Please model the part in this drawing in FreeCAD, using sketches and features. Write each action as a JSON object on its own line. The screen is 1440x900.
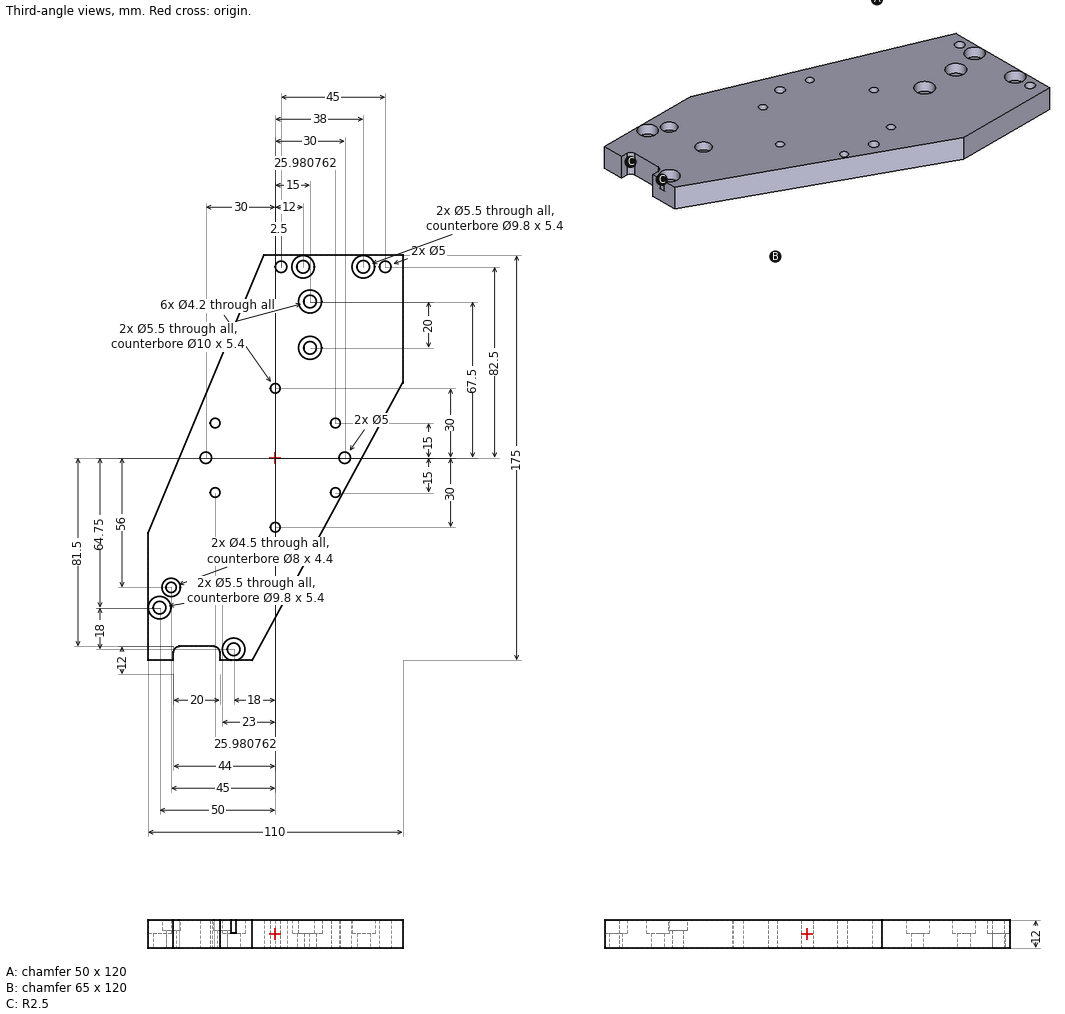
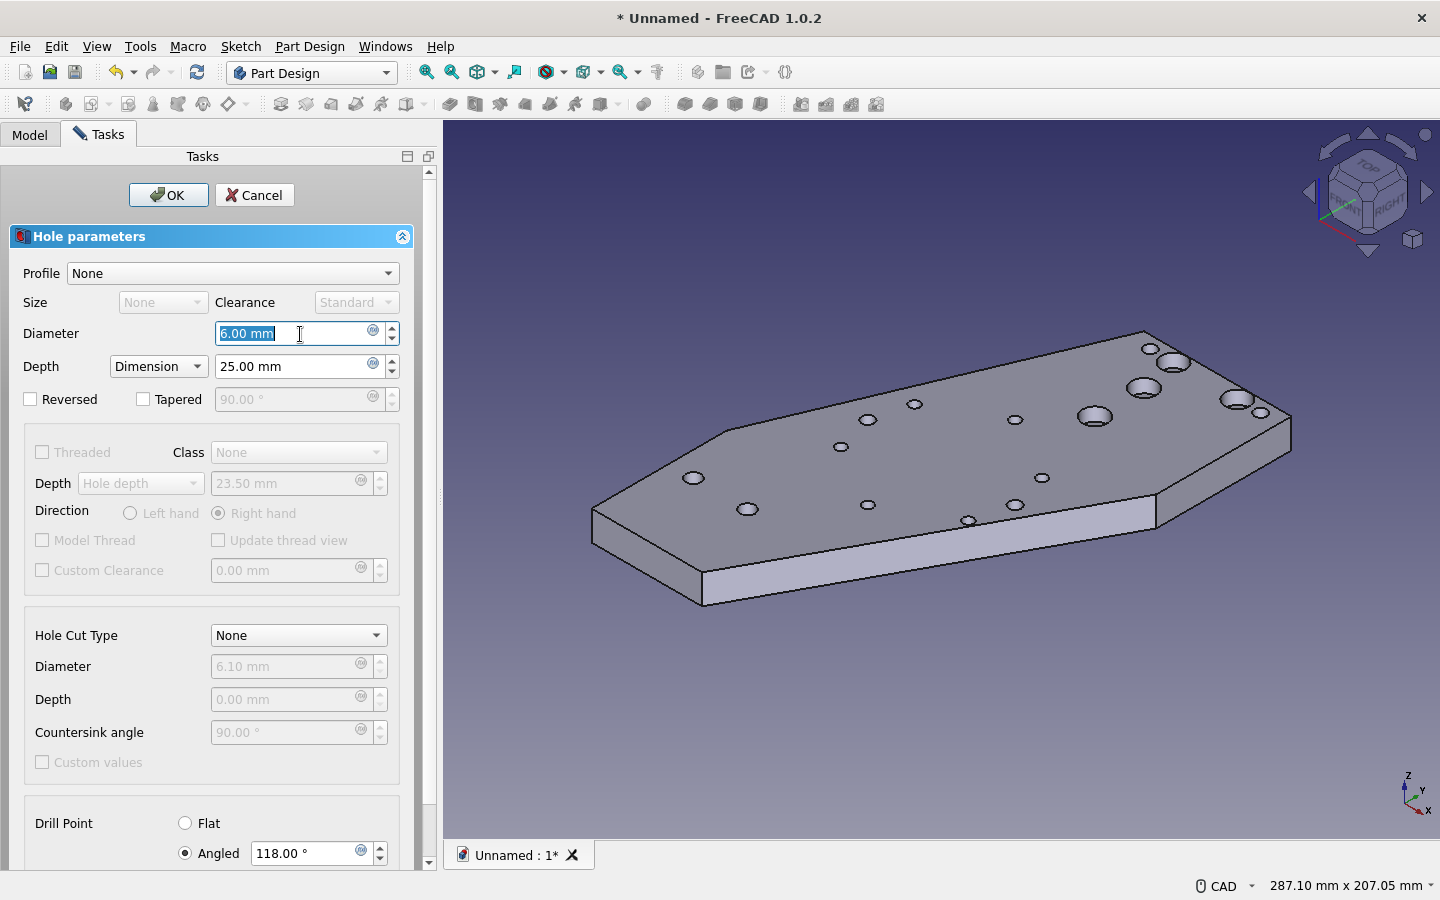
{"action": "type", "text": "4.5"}
{"action": "key", "text": "Tab"}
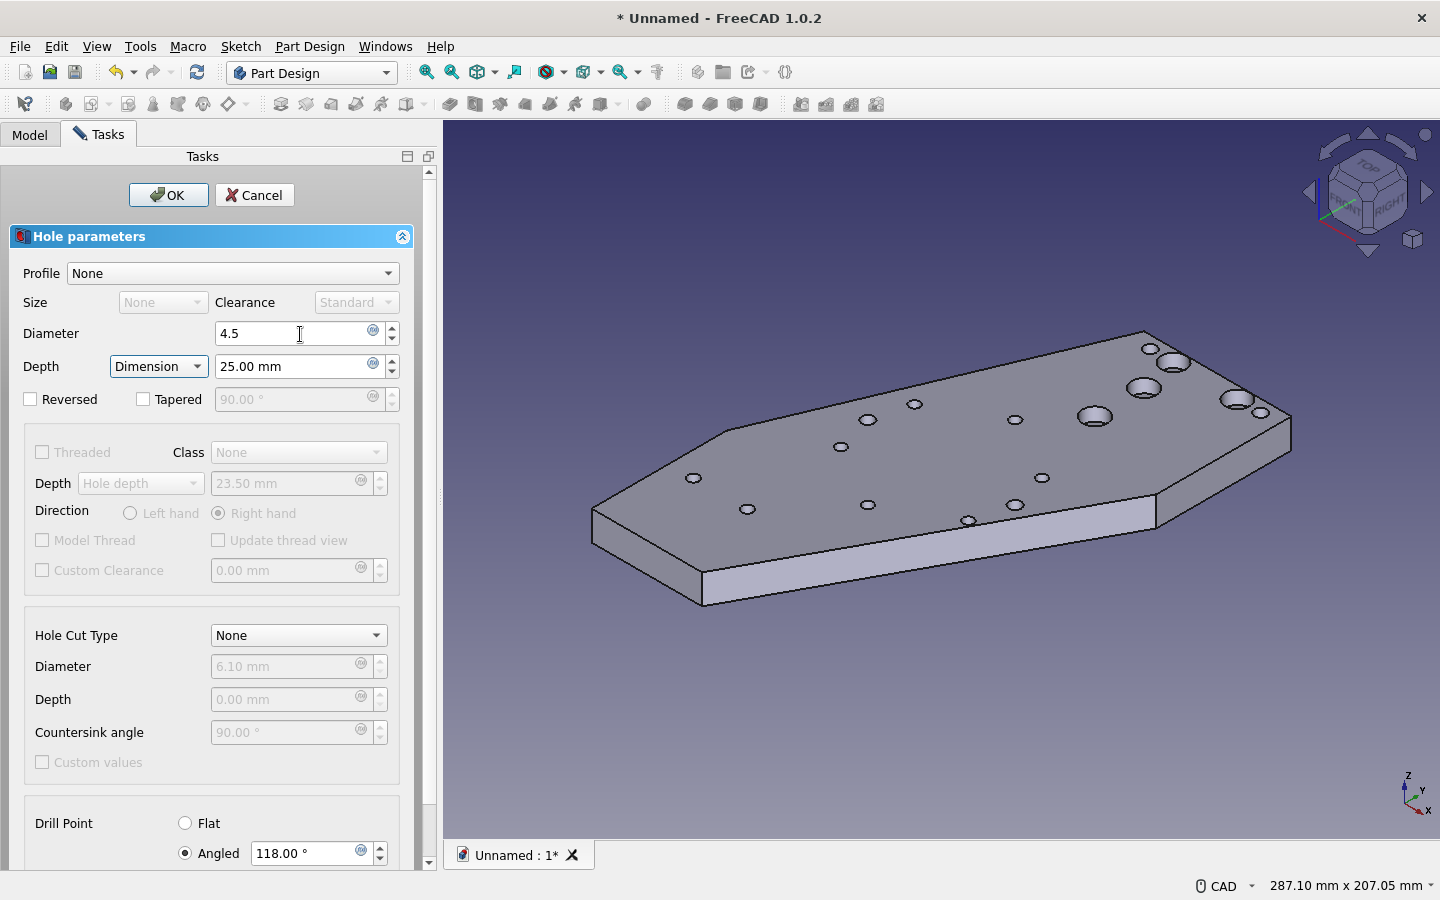
{"action": "left_click", "coordinate": [160, 366]}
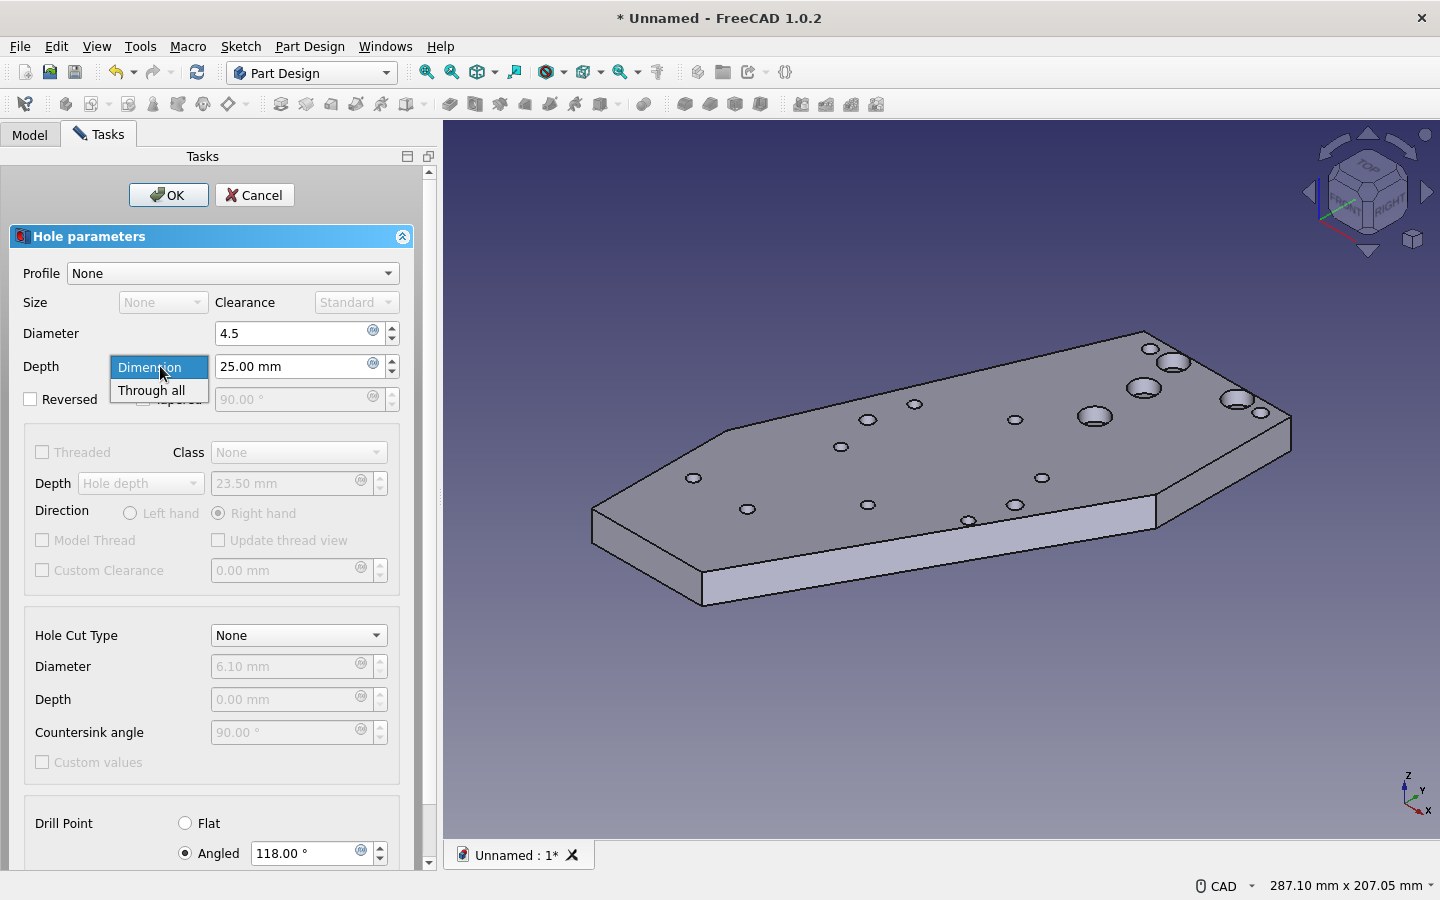
{"action": "left_click", "coordinate": [158, 390]}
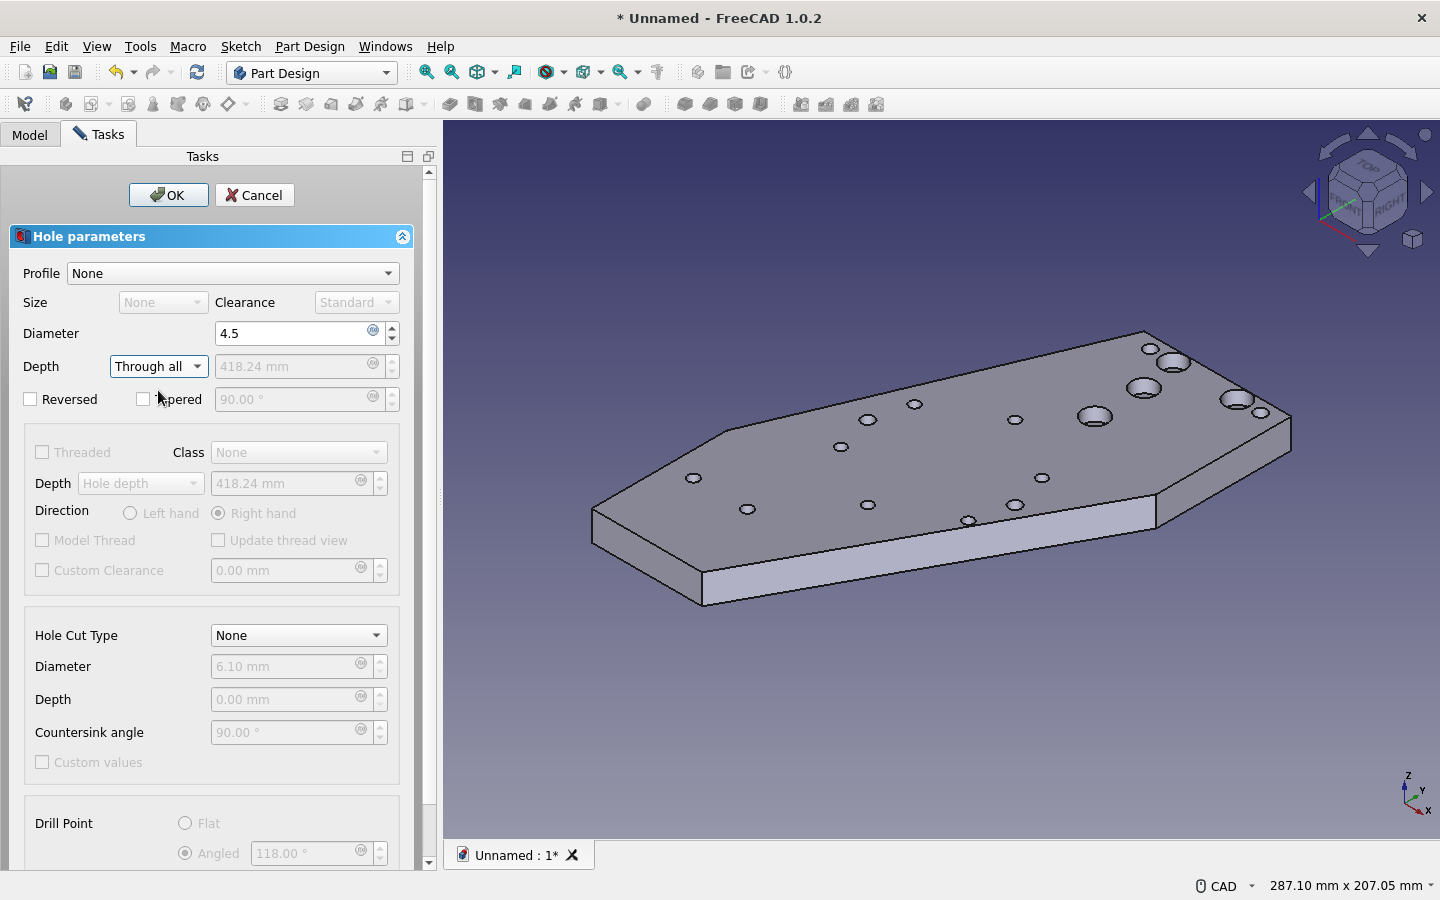
{"action": "left_click", "coordinate": [300, 636]}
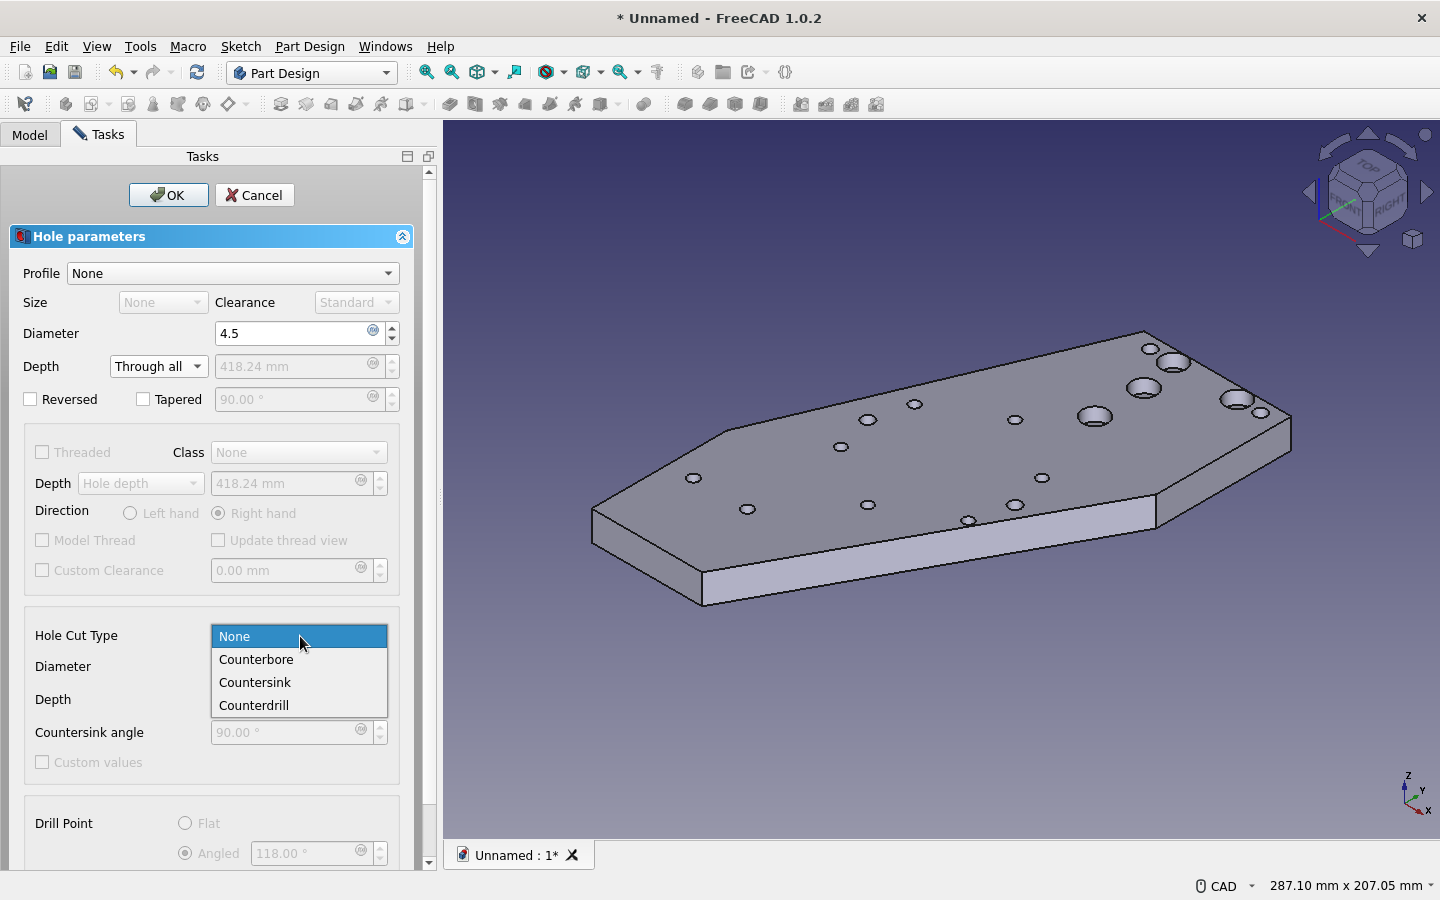
{"action": "left_click", "coordinate": [298, 660]}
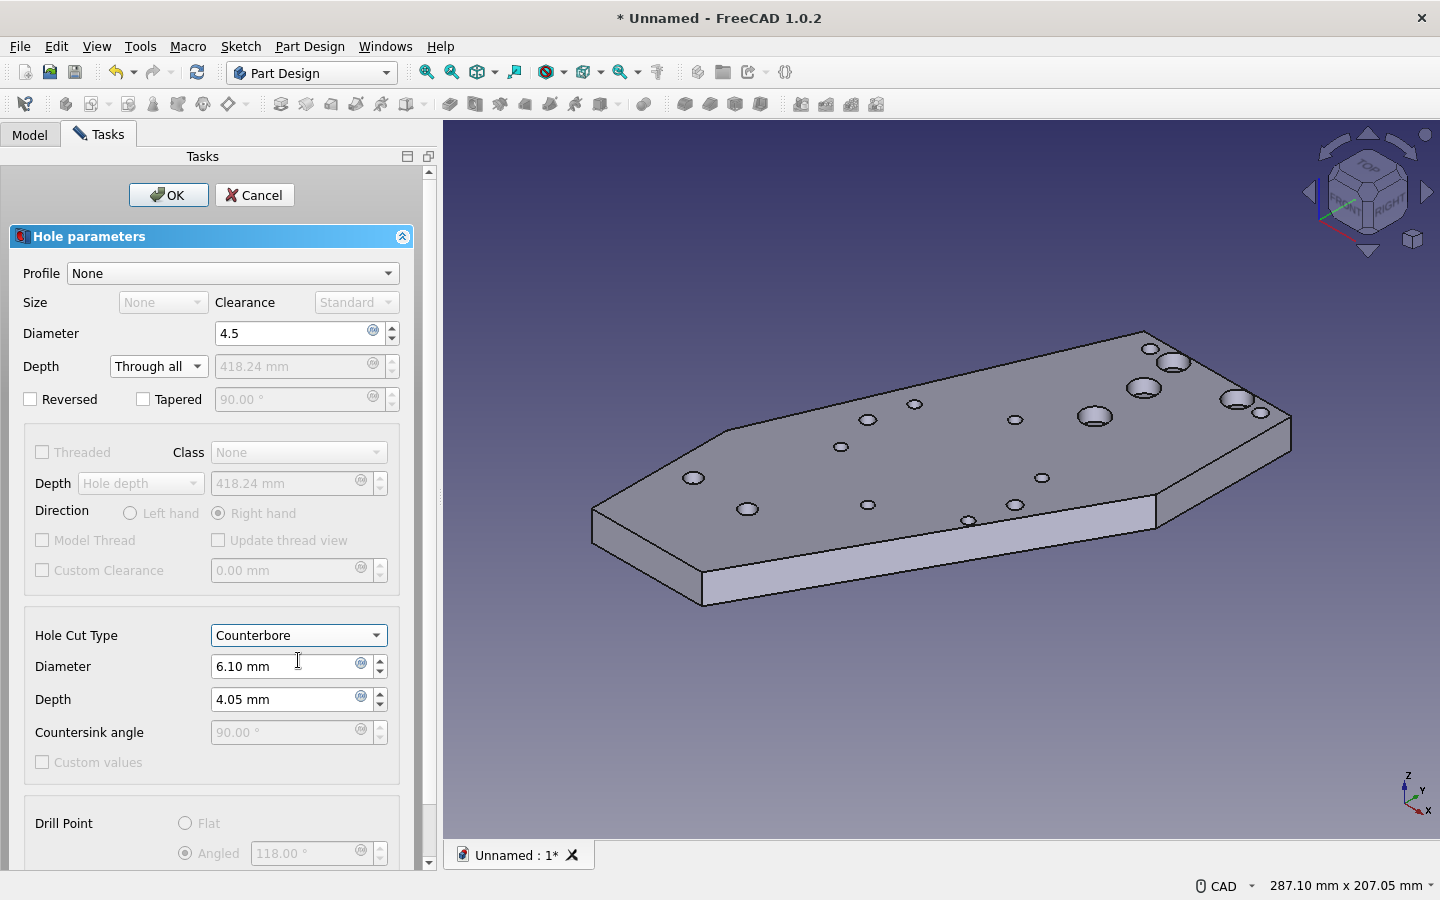
{"action": "triple_click", "coordinate": [292, 666]}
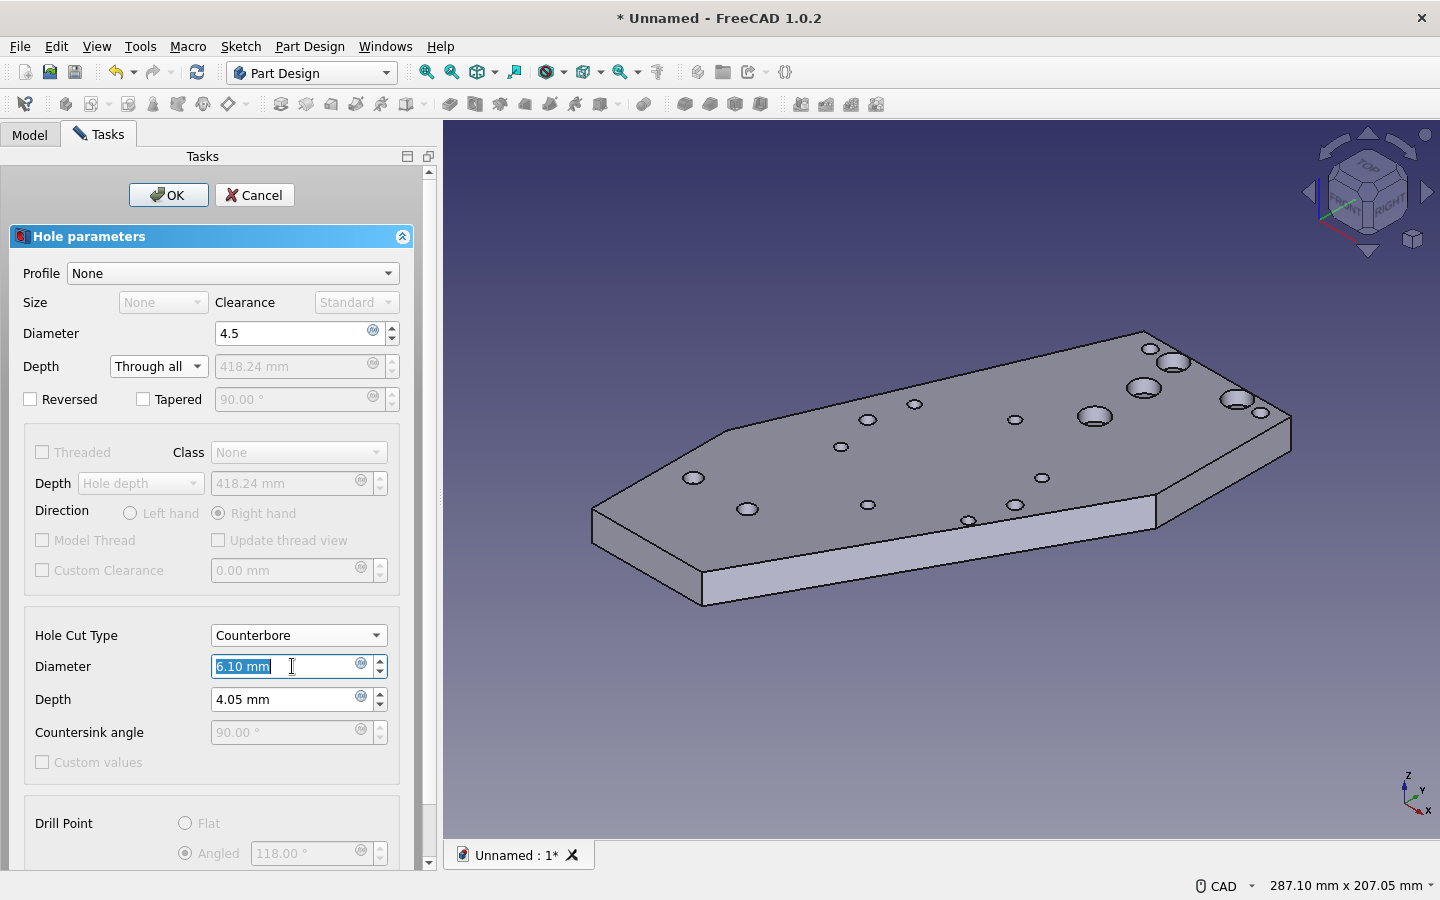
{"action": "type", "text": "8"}
{"action": "key", "text": "Tab"}